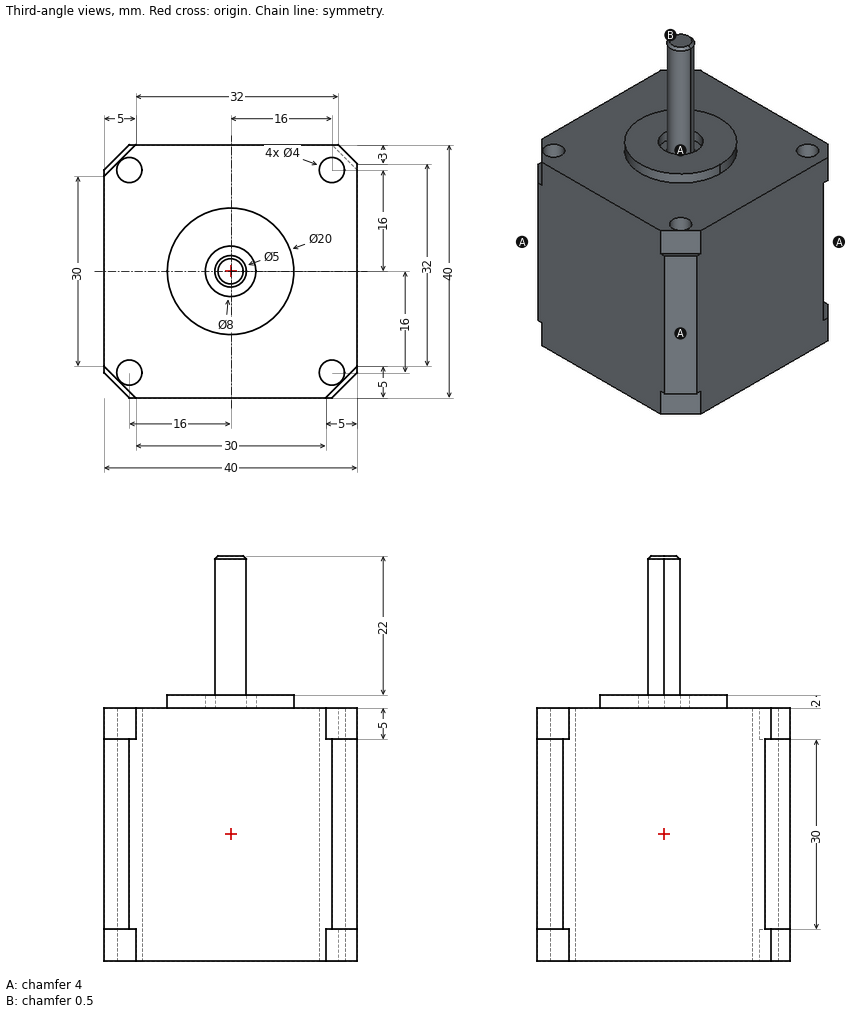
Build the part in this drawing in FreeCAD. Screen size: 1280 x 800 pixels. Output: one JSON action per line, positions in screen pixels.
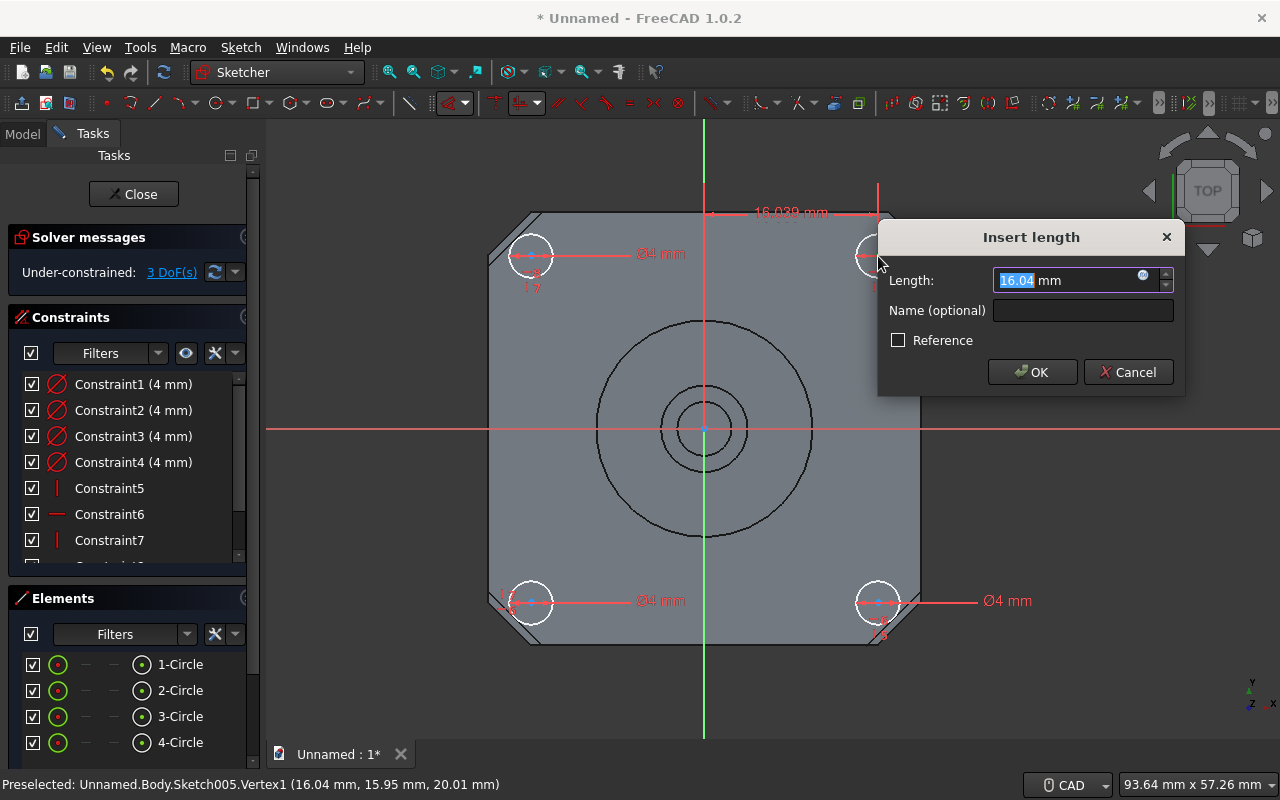
{"action": "type", "text": "16"}
{"action": "key", "text": "Return"}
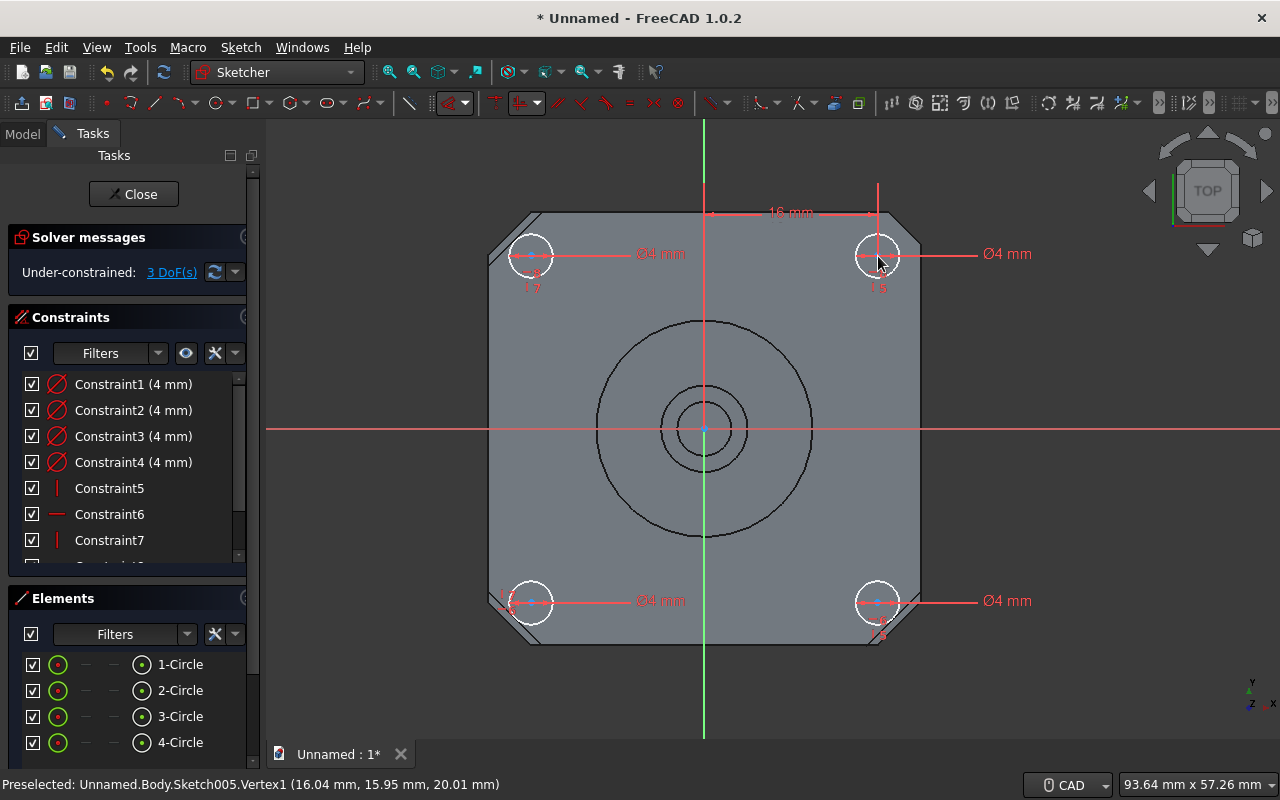
{"action": "left_click", "coordinate": [878, 256]}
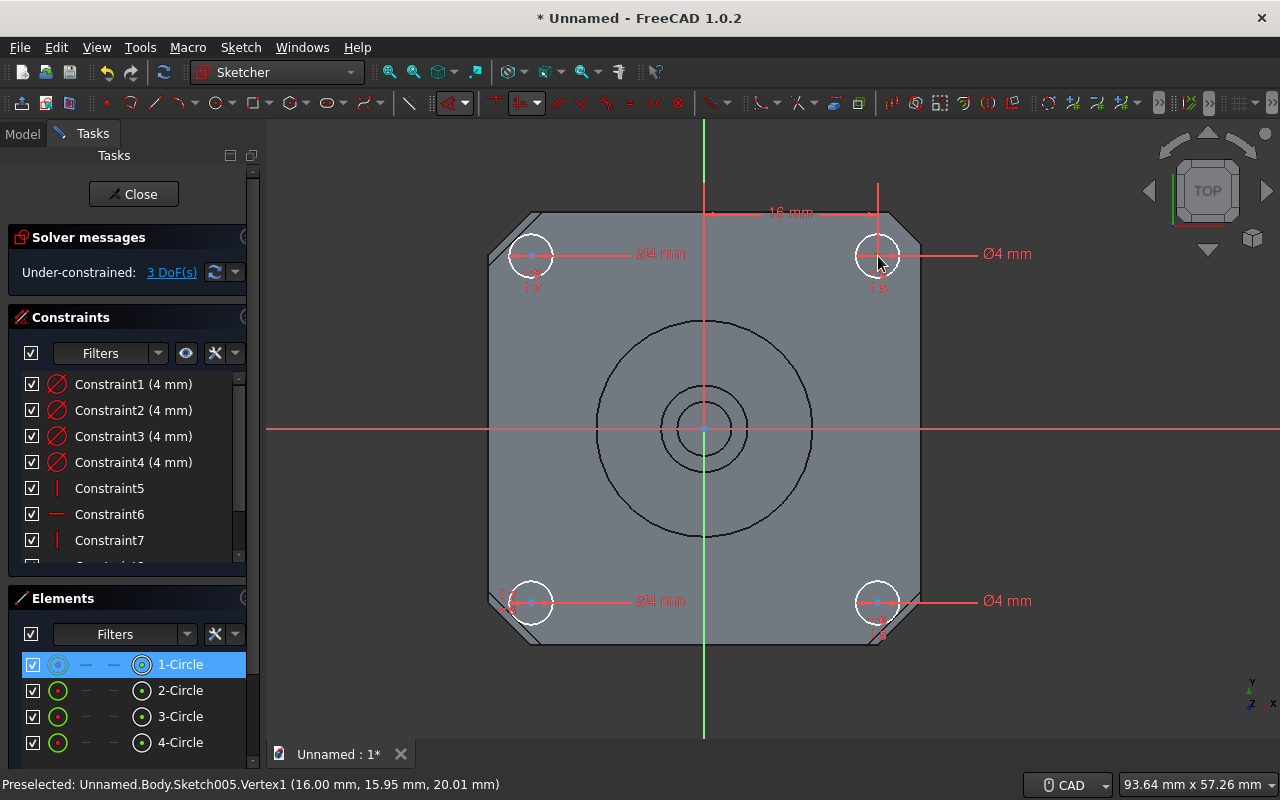
{"action": "key", "text": "i"}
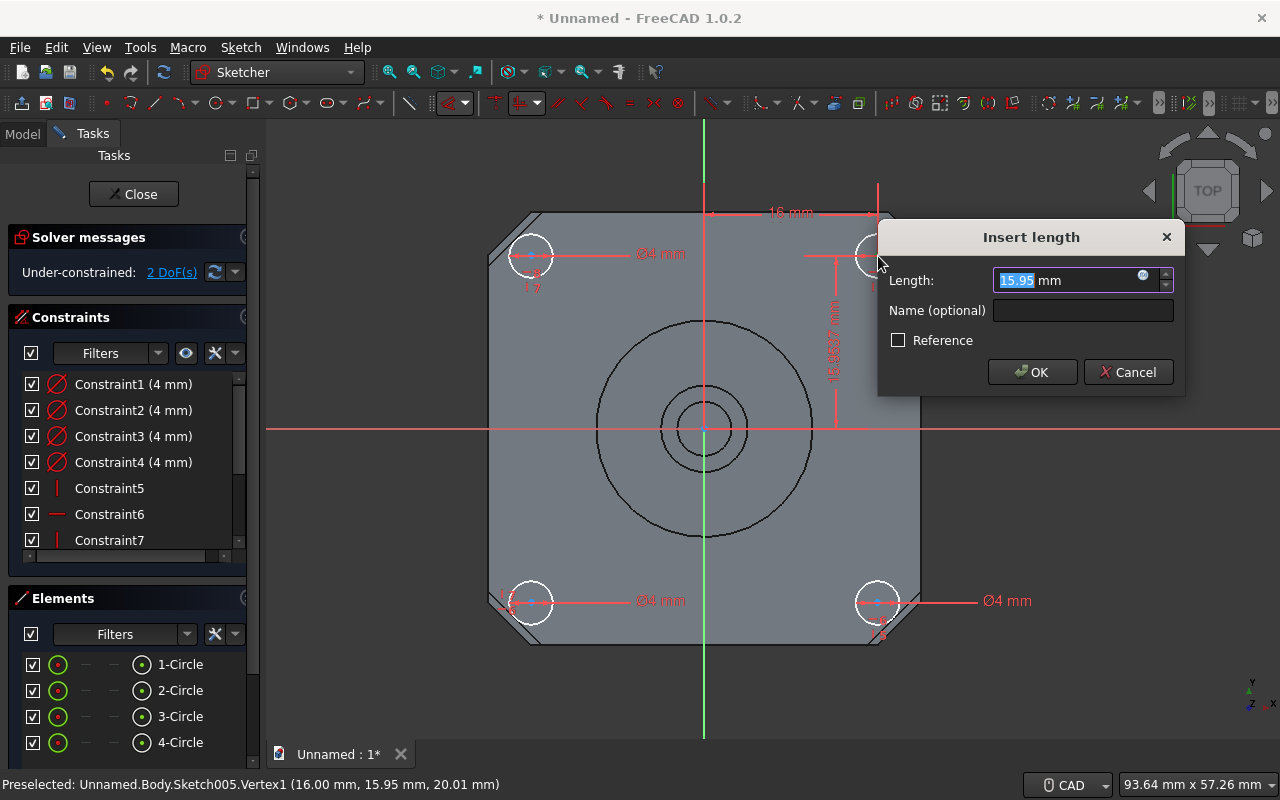
{"action": "type", "text": "16"}
{"action": "key", "text": "Return"}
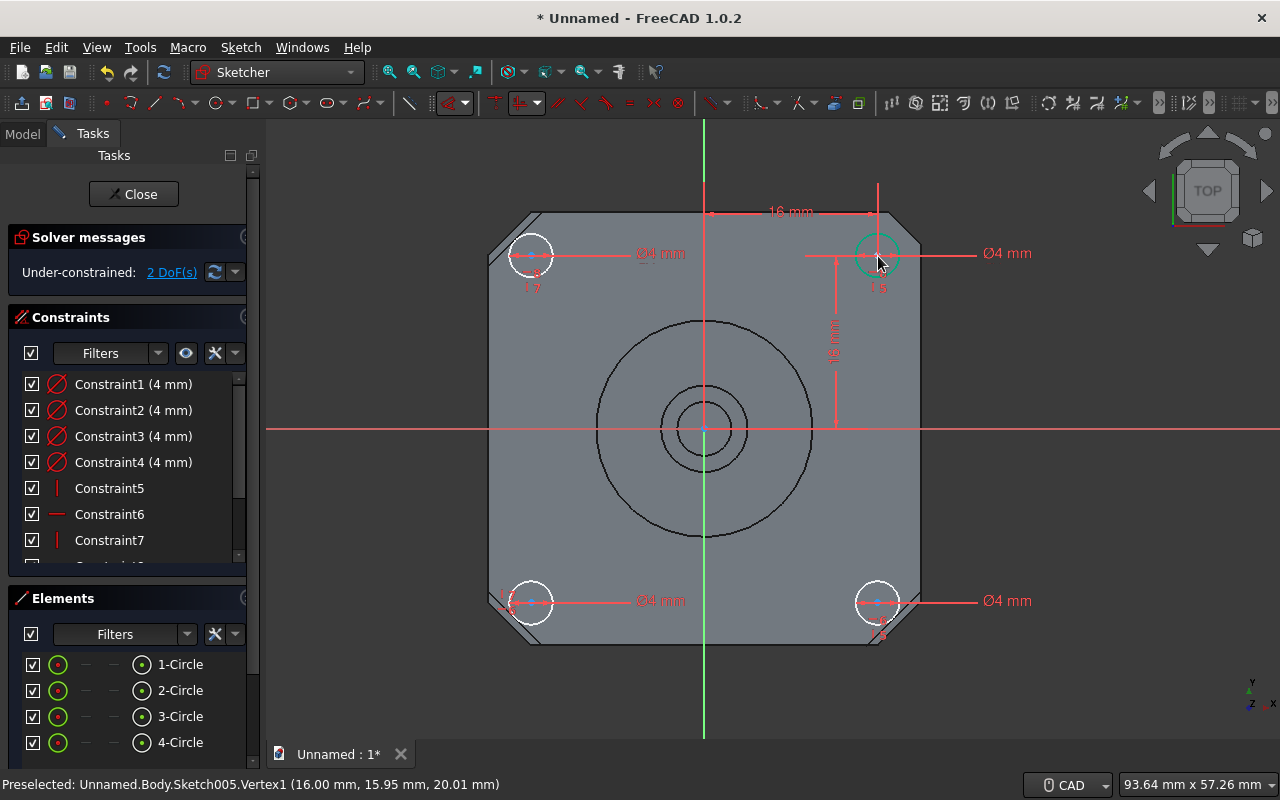
{"action": "left_click", "coordinate": [878, 603]}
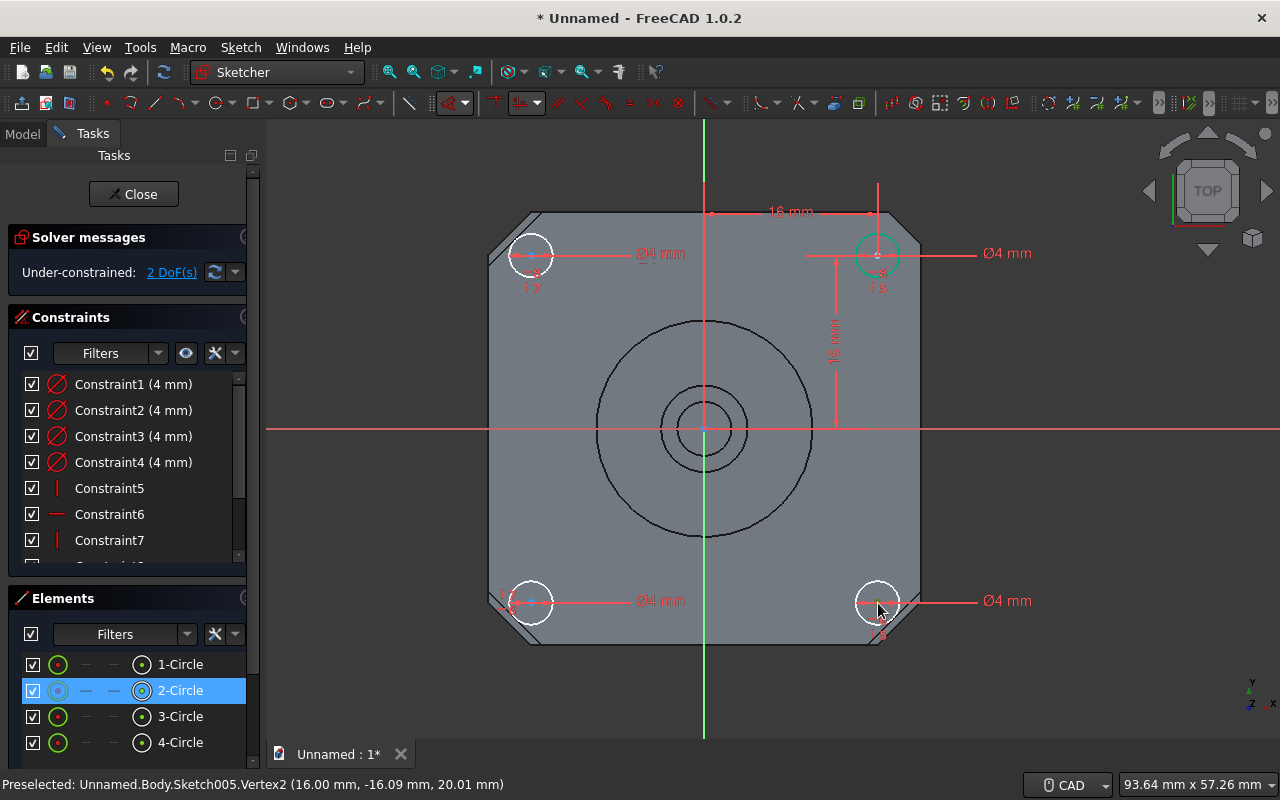
{"action": "left_click", "coordinate": [468, 104]}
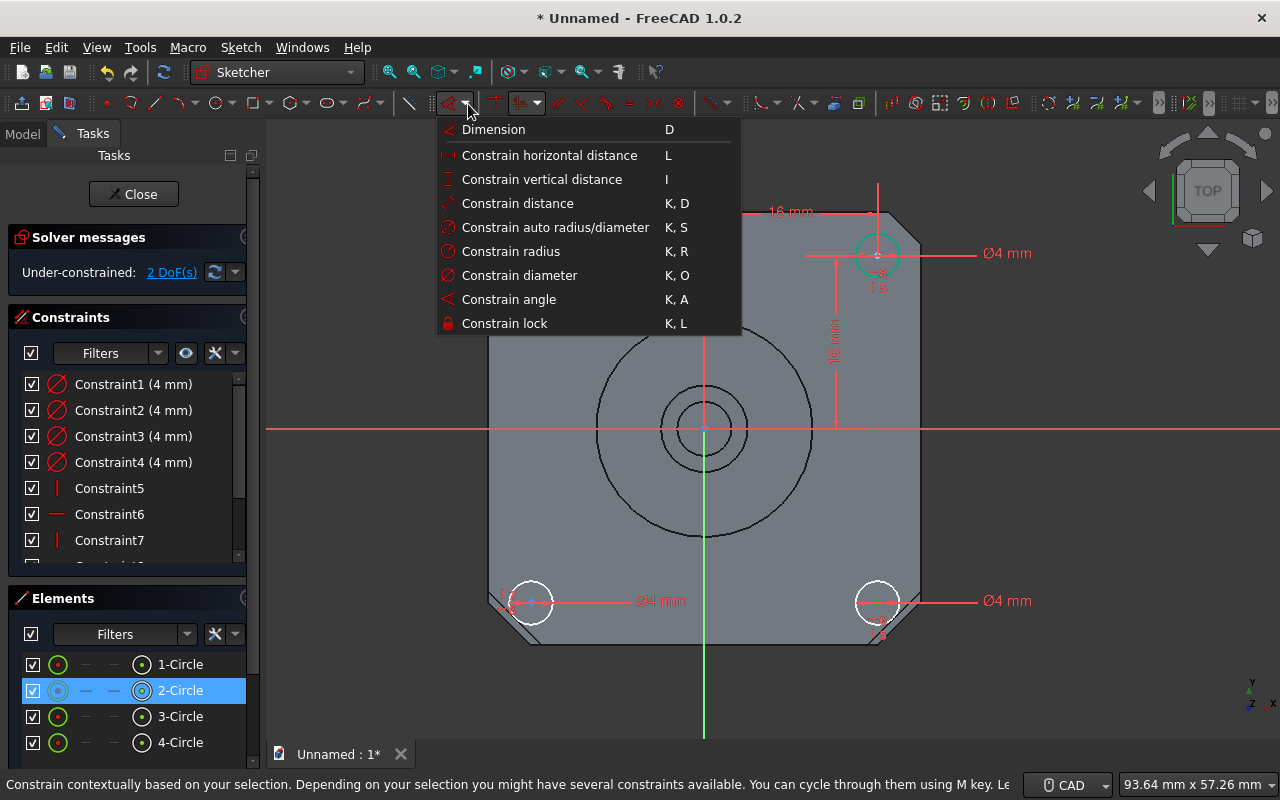
{"action": "left_click", "coordinate": [589, 179]}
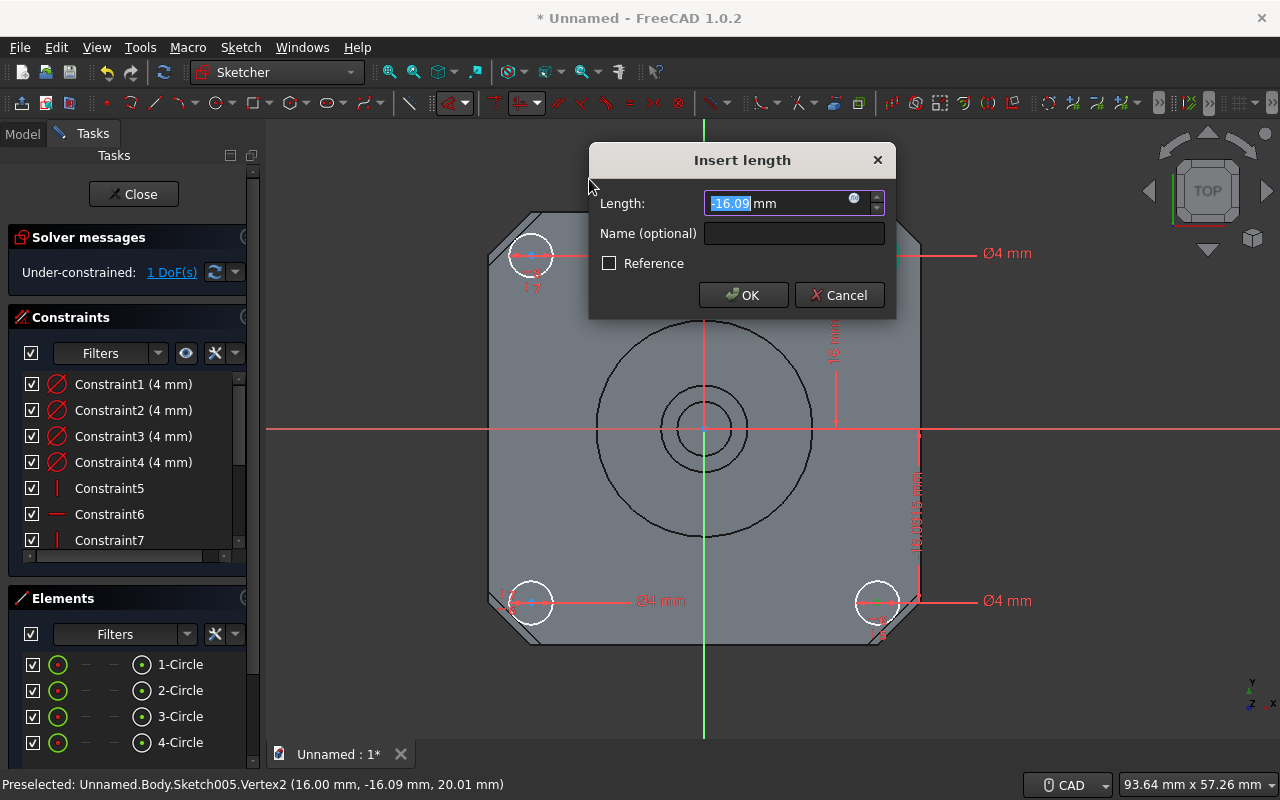
{"action": "type", "text": "-16"}
{"action": "key", "text": "Return"}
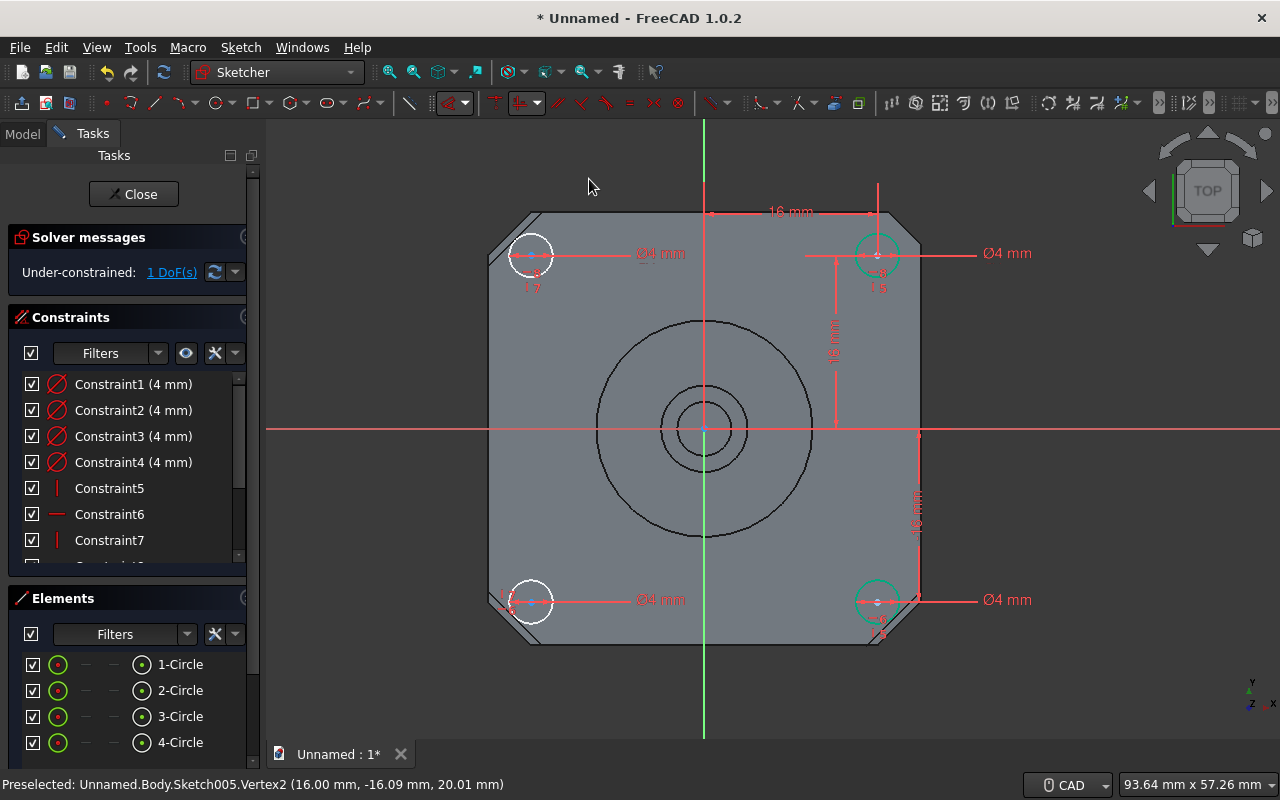
{"action": "left_click", "coordinate": [531, 602]}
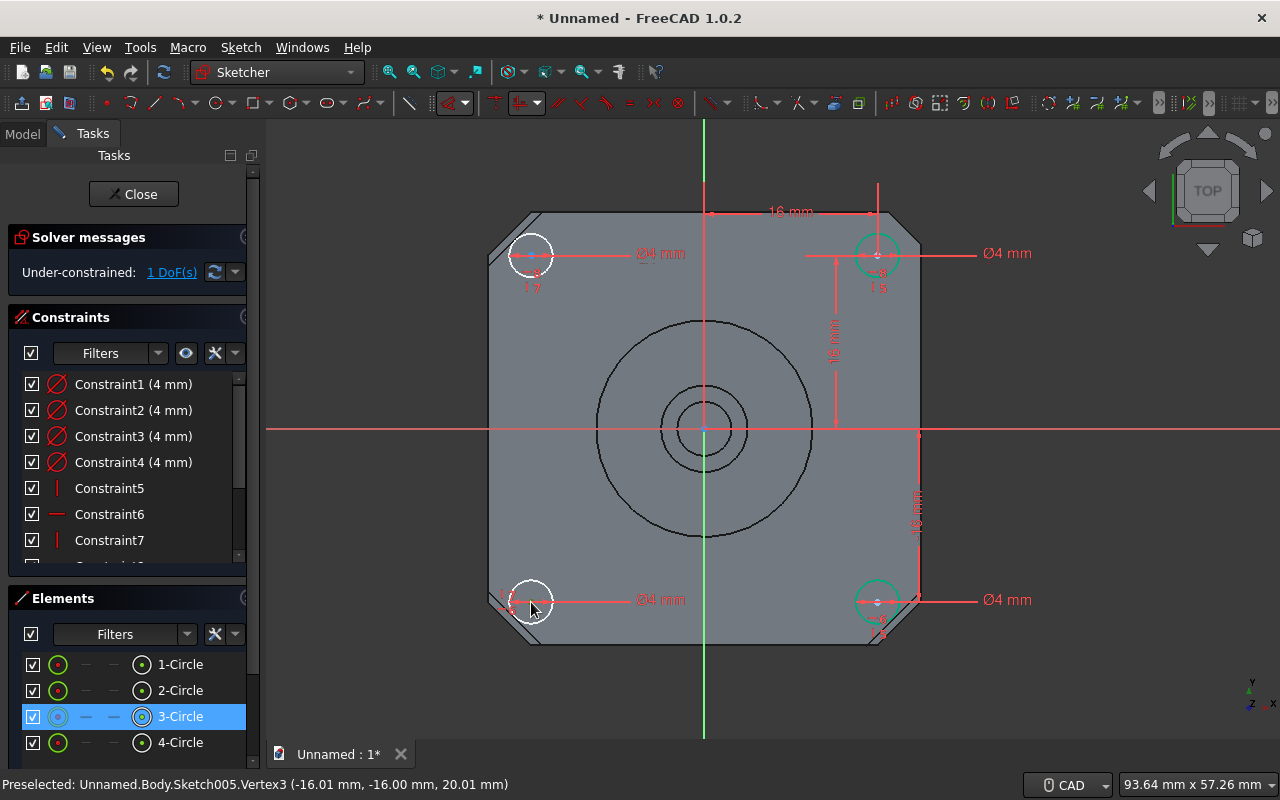
{"action": "key", "text": "l"}